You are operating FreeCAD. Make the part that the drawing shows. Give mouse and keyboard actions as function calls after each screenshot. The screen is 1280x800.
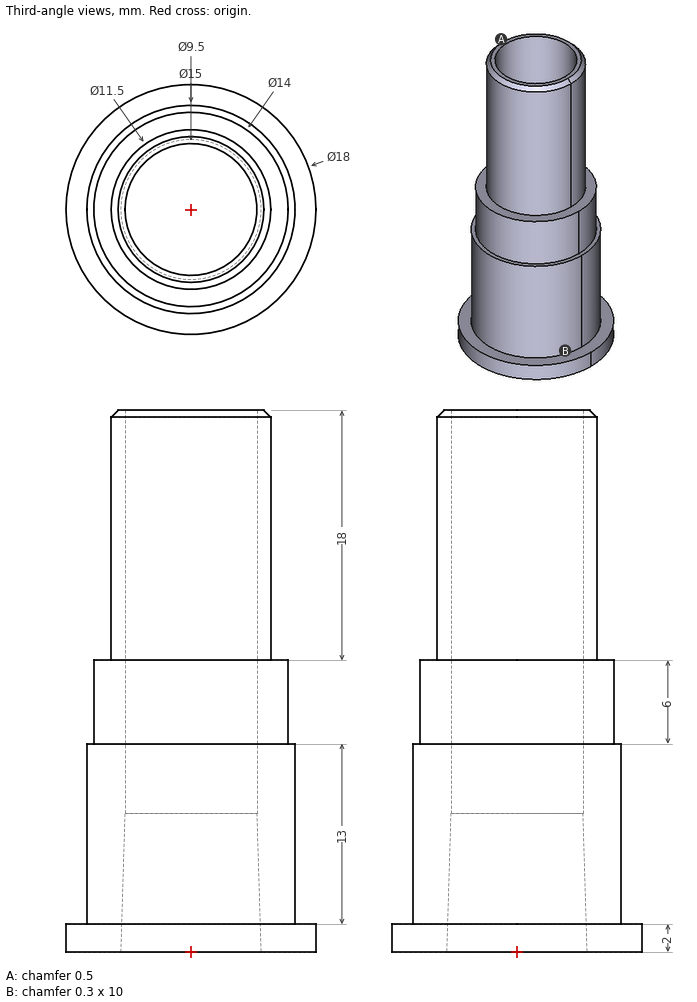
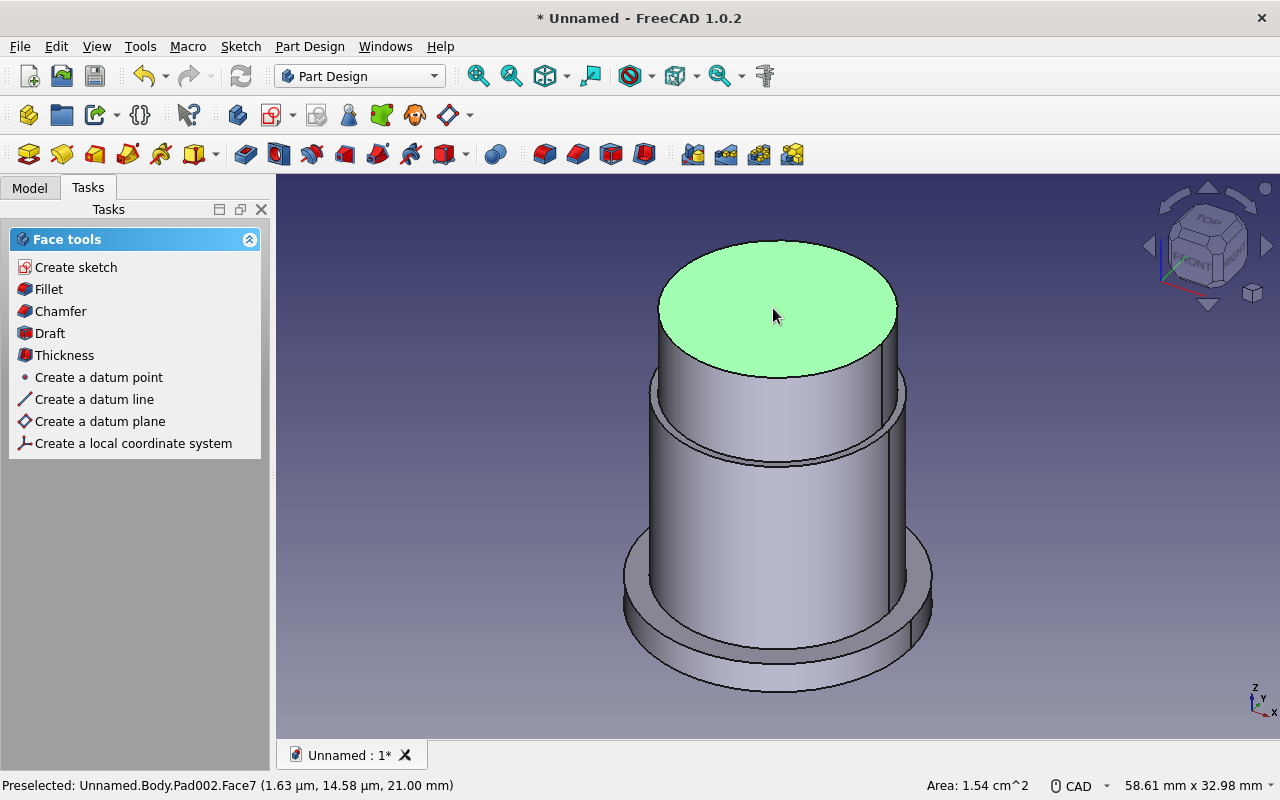
click(270, 116)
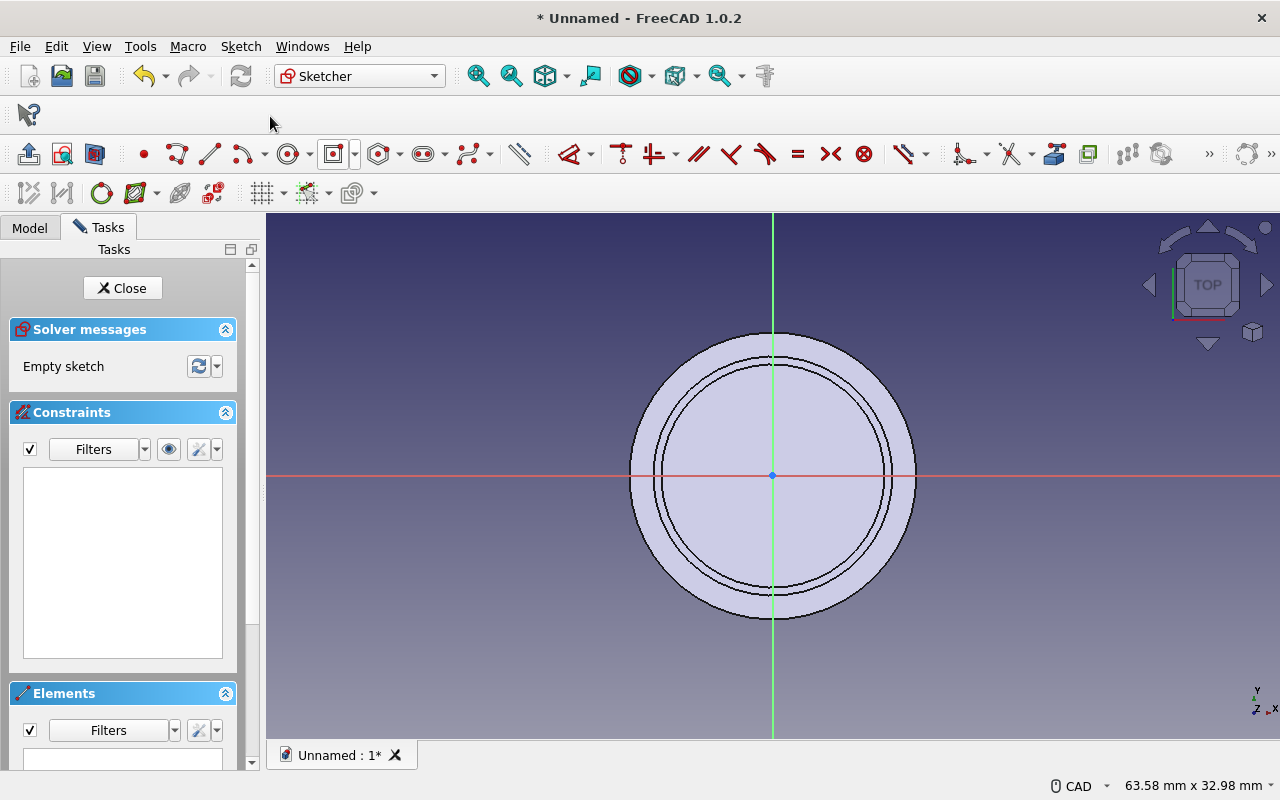
scroll(856, 476, up, 3)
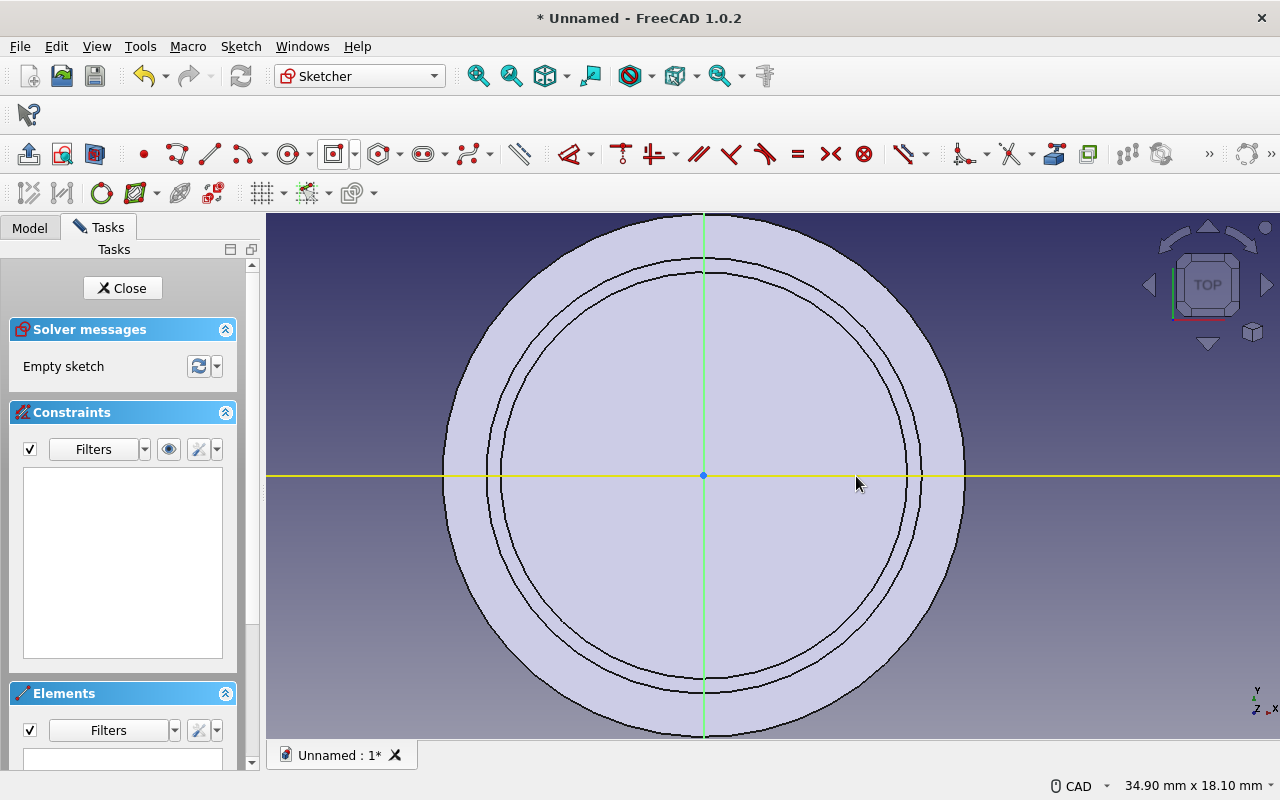
click(288, 154)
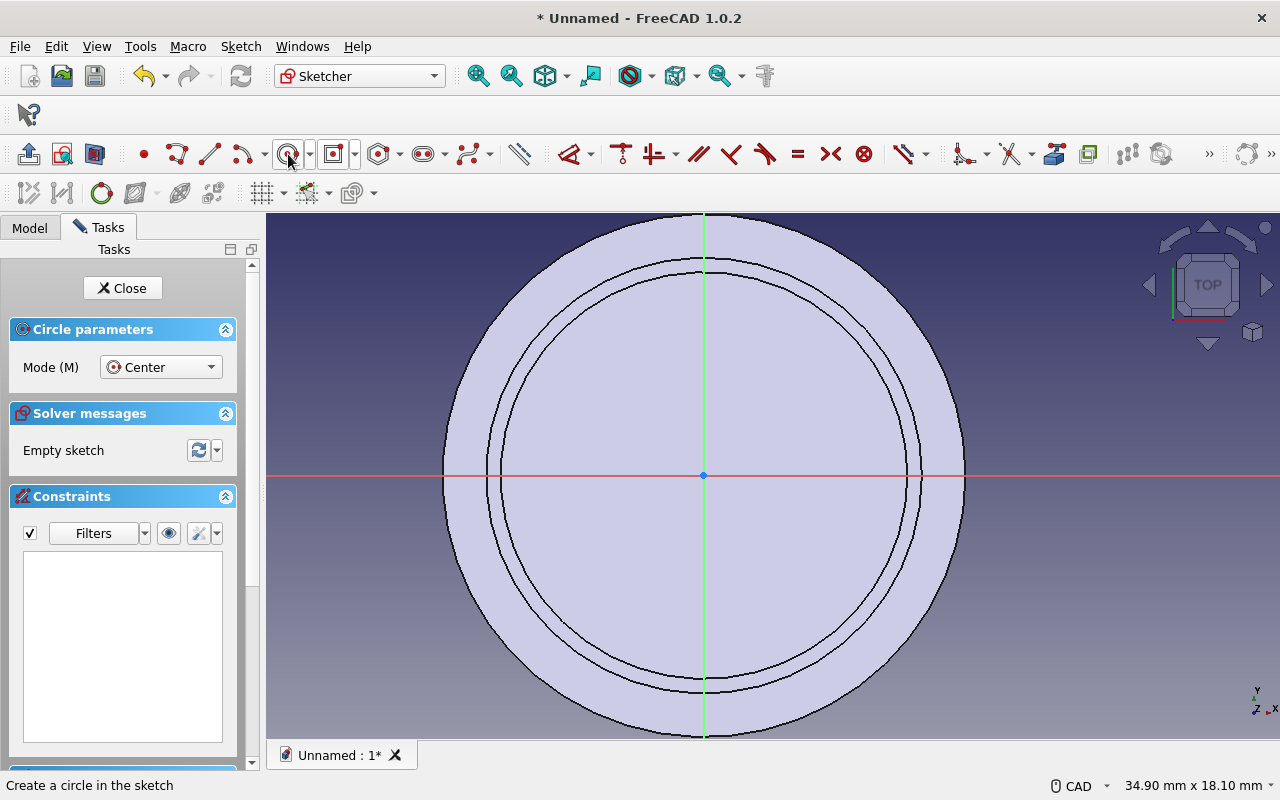
click(704, 476)
click(822, 357)
key(Escape)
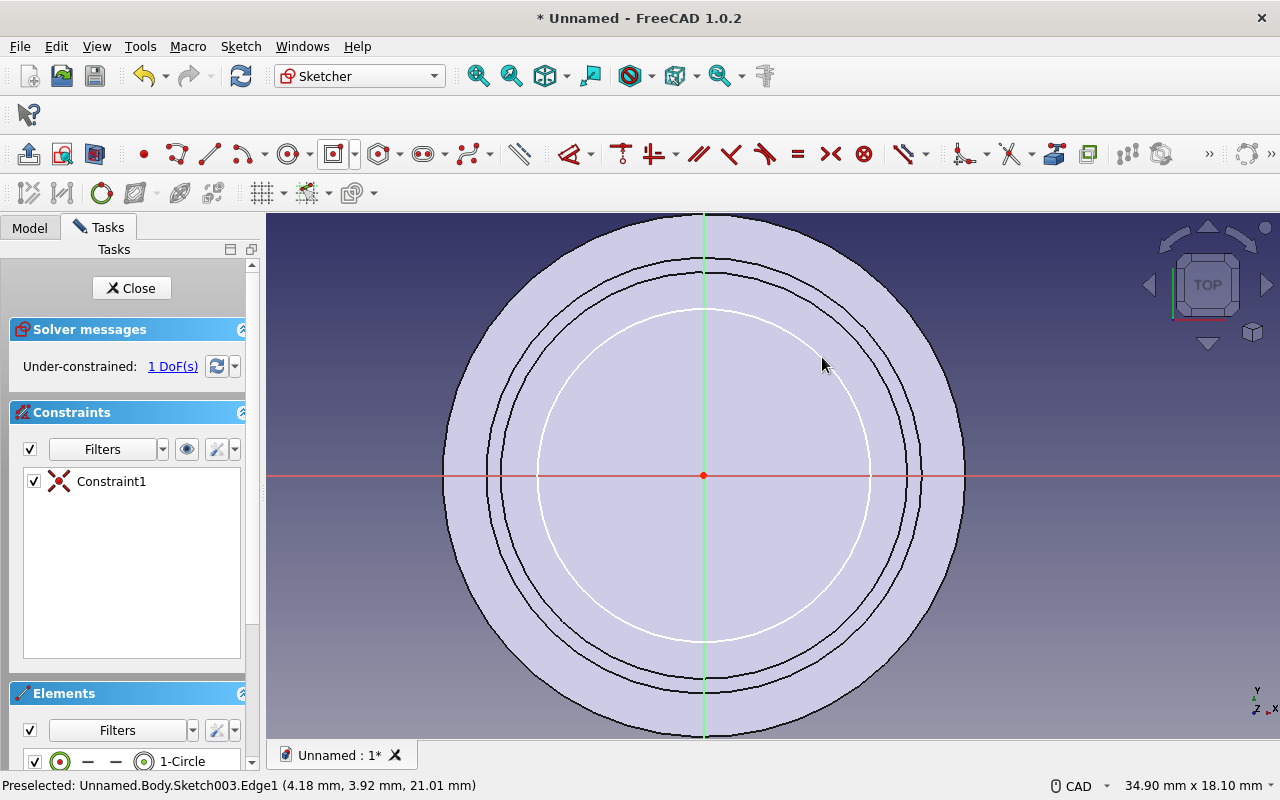
click(568, 154)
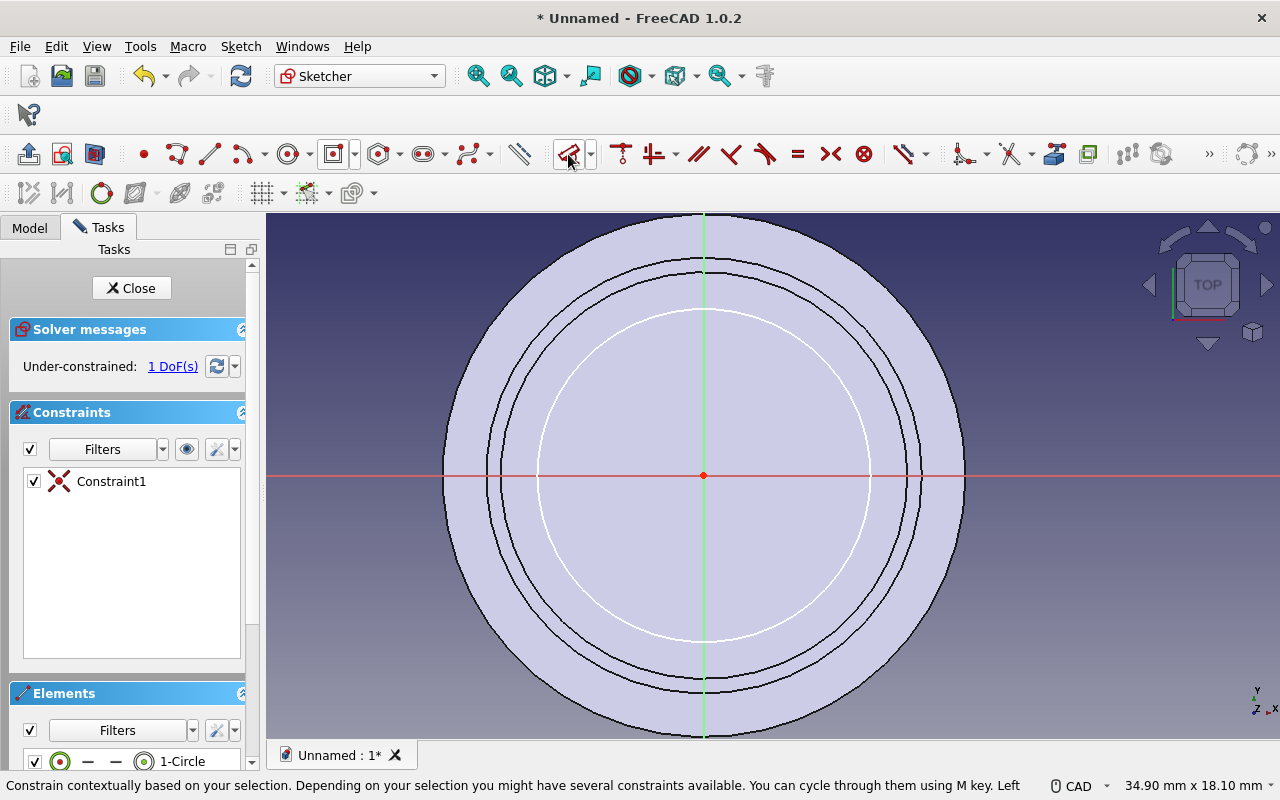
click(821, 357)
click(843, 334)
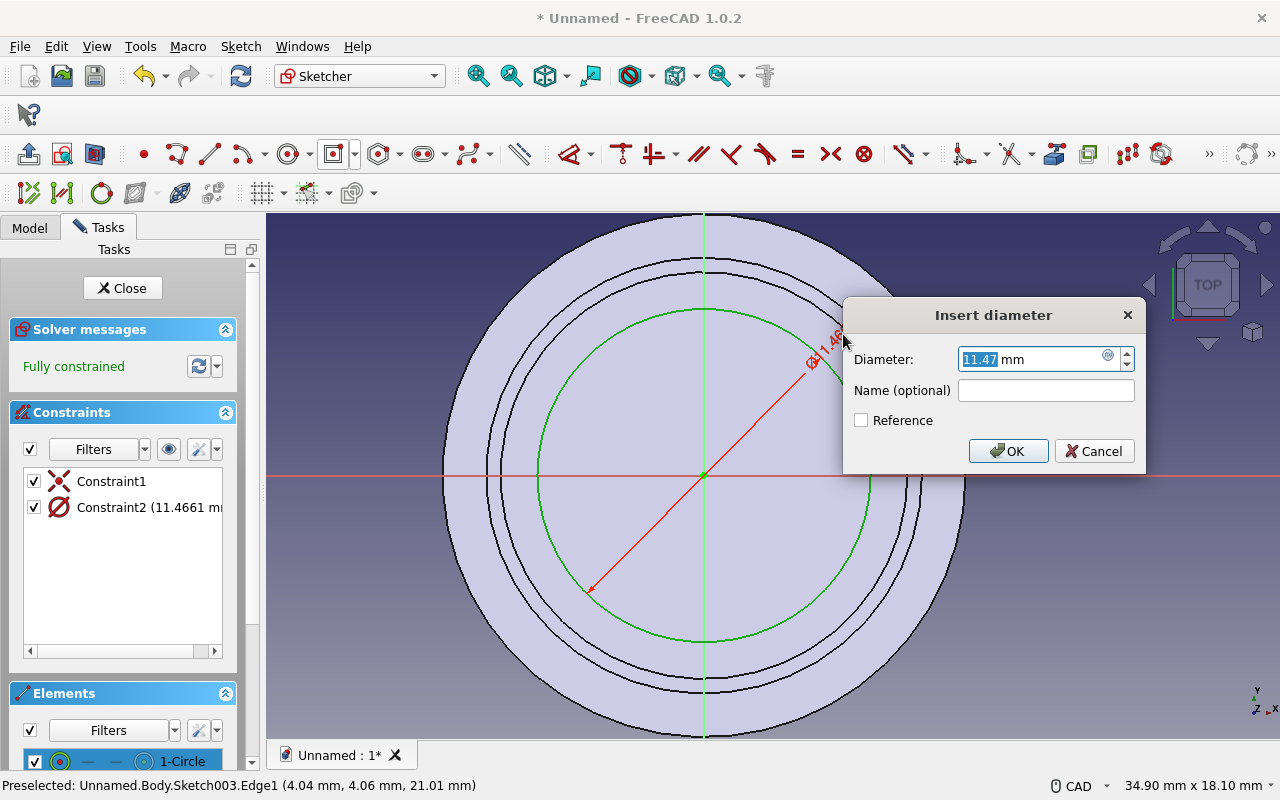
text(11.5)
key(Return)
key(Escape)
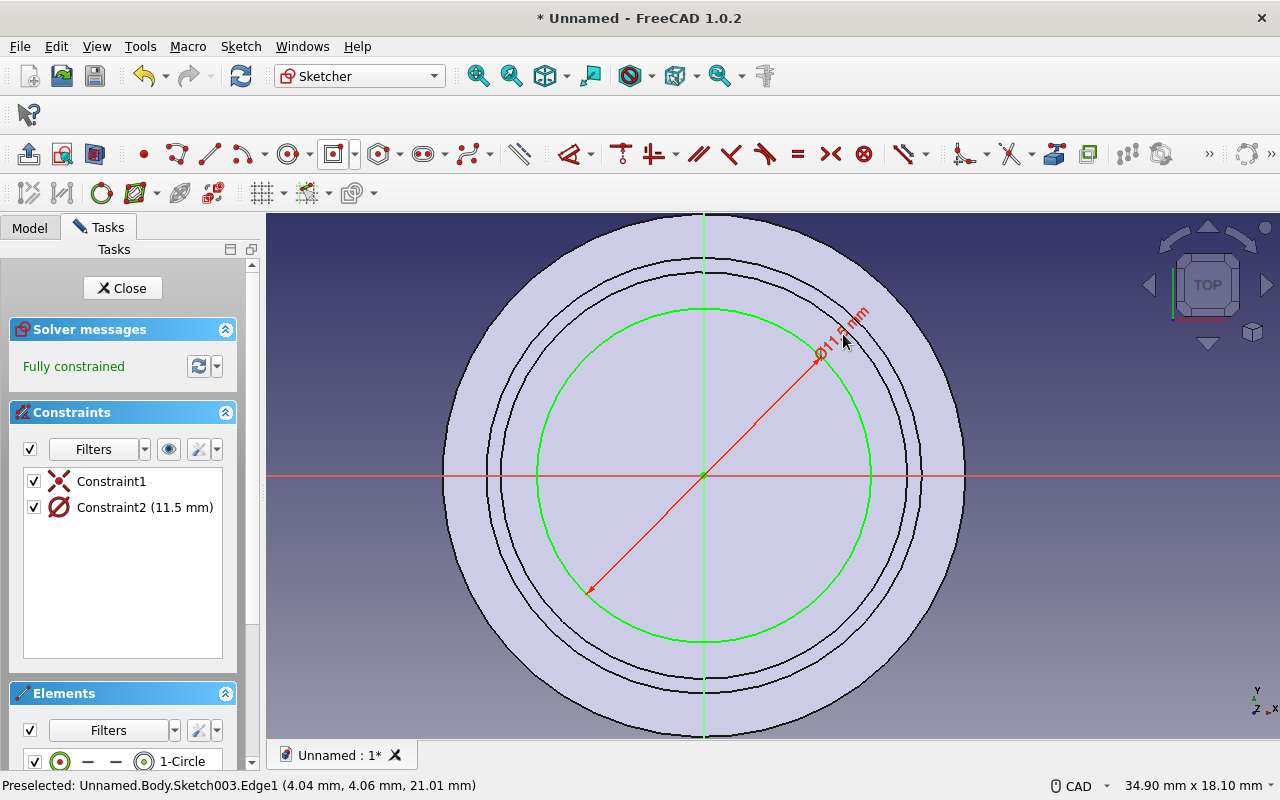
click(123, 288)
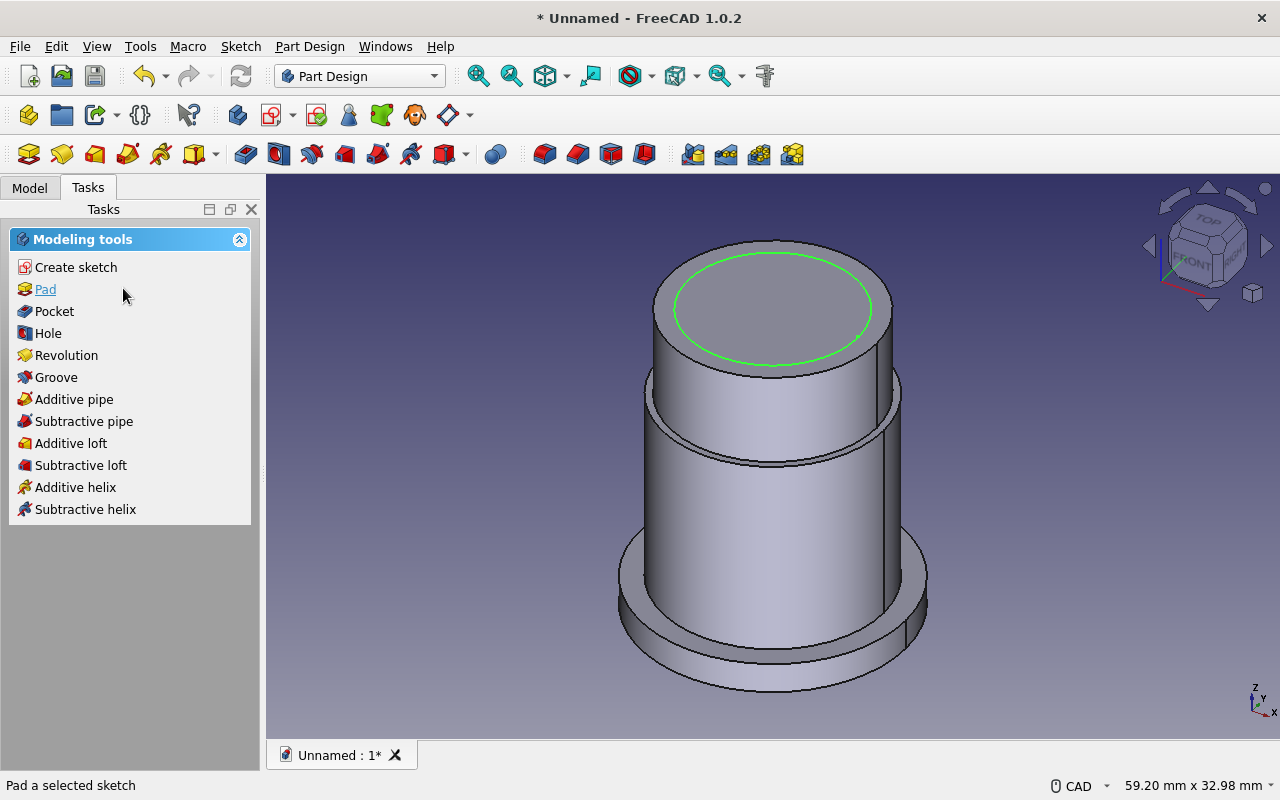
click(29, 154)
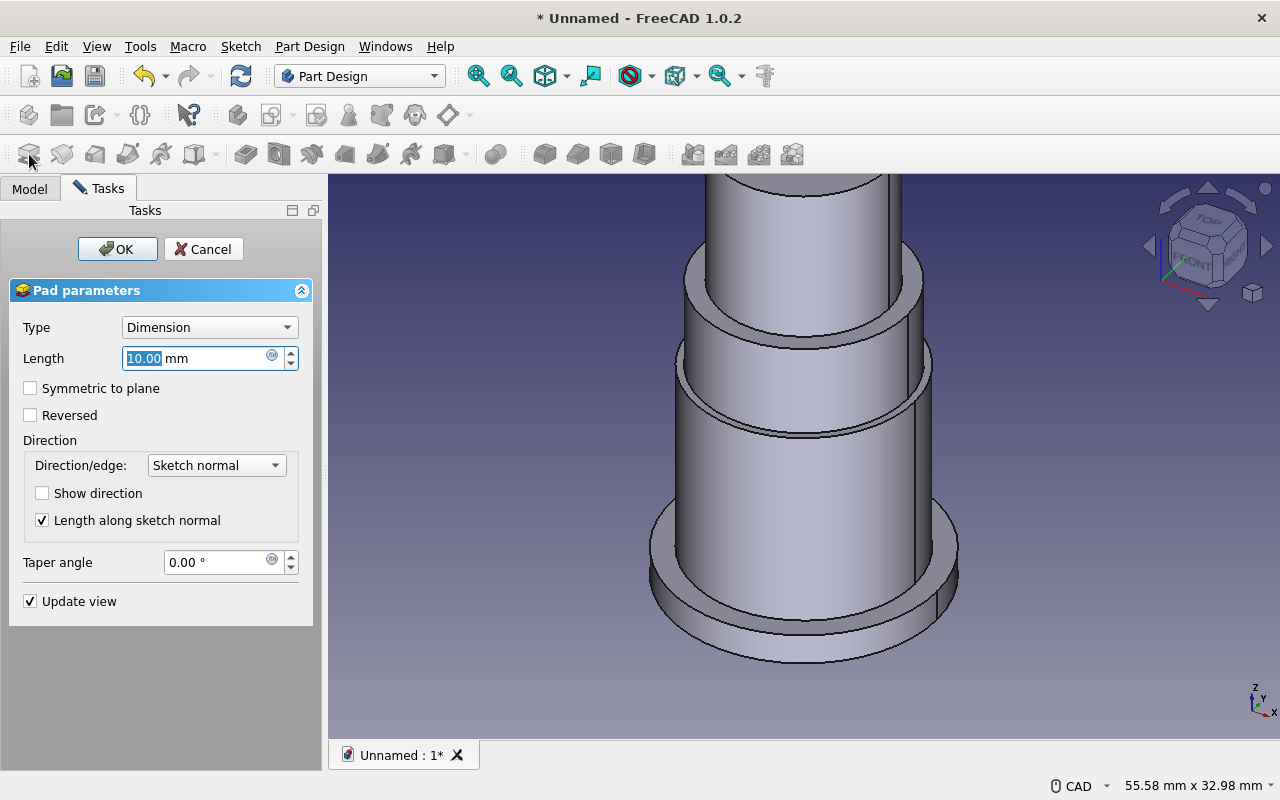
text(18)
key(Tab)